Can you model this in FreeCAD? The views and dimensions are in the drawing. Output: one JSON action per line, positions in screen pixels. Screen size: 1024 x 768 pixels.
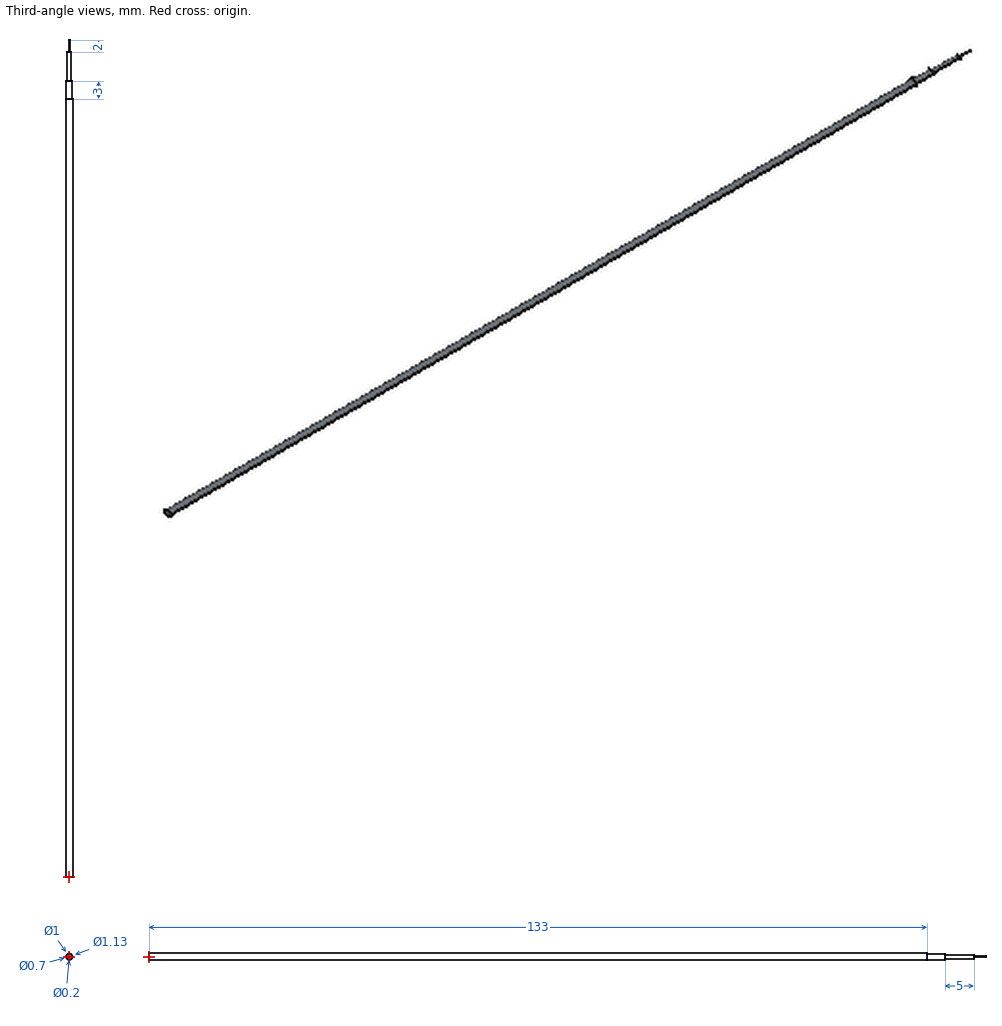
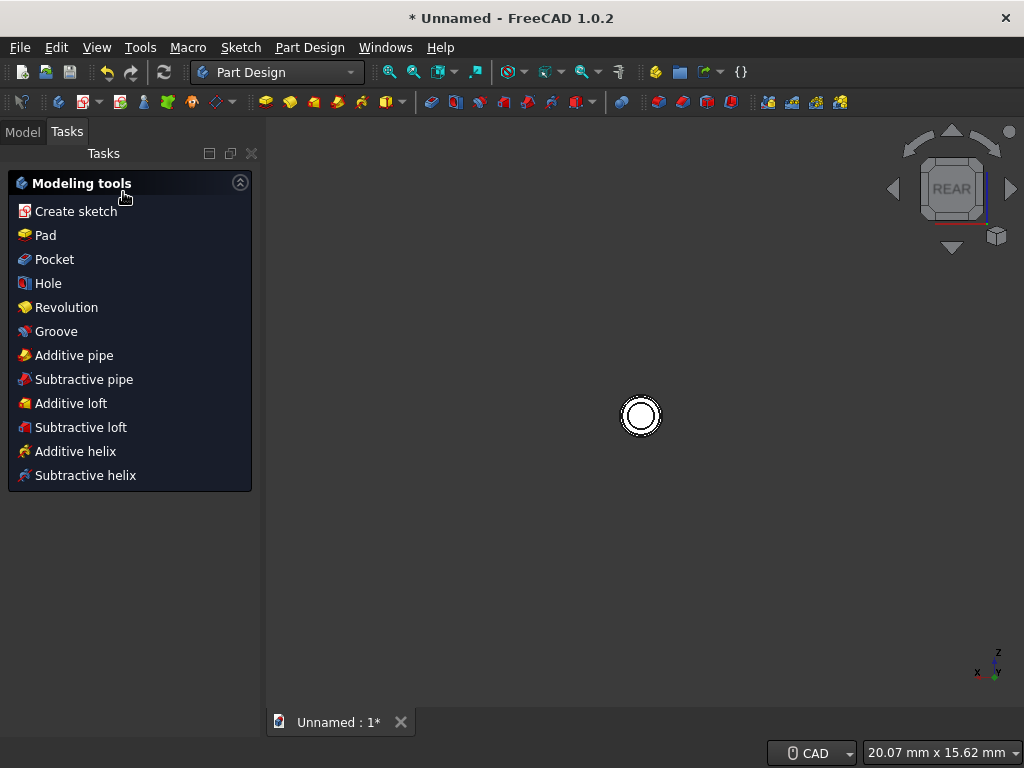
{"action": "left_click", "coordinate": [266, 102]}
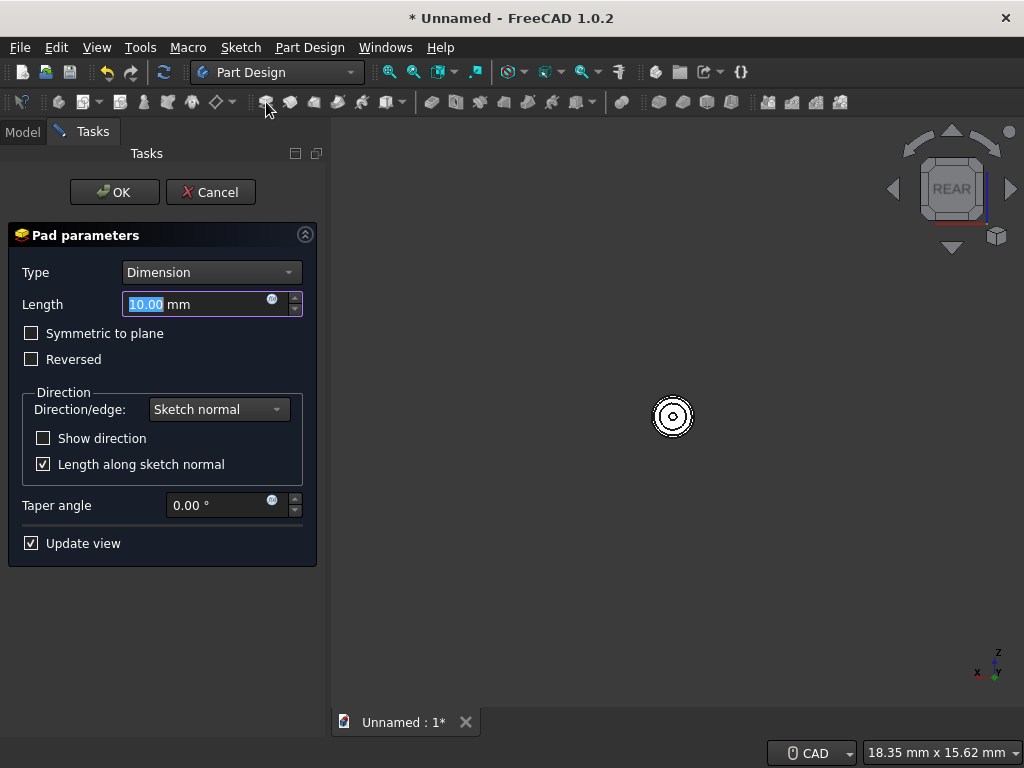
{"action": "type", "text": "2"}
{"action": "key", "text": "Tab"}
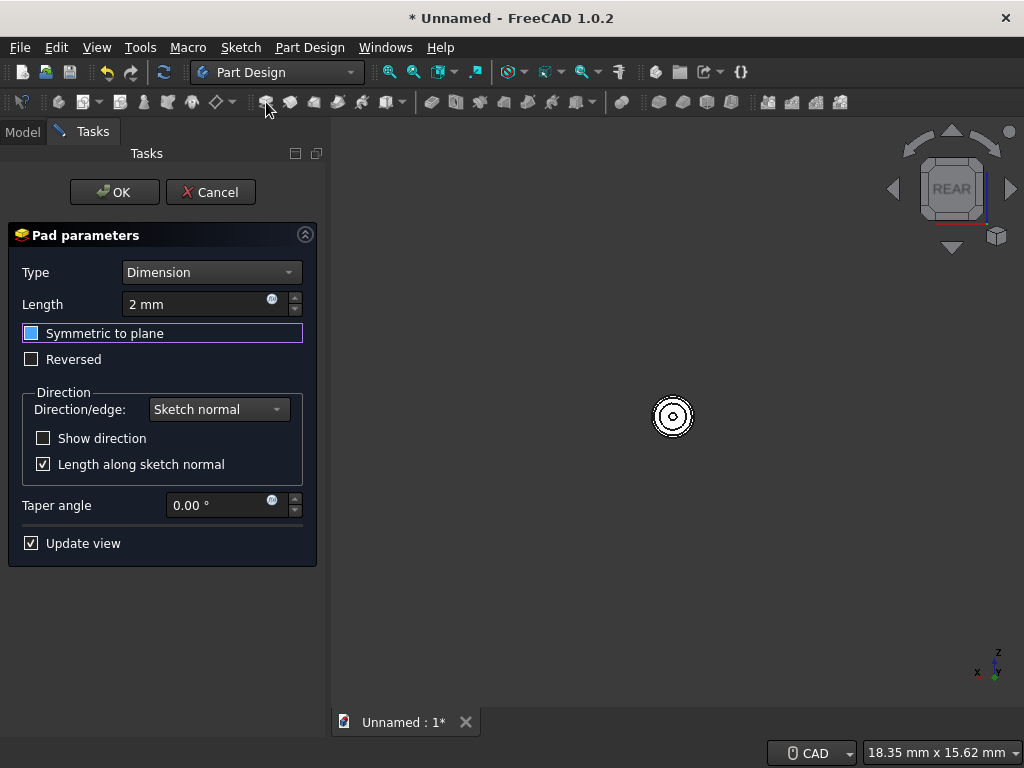
{"action": "left_click", "coordinate": [115, 192]}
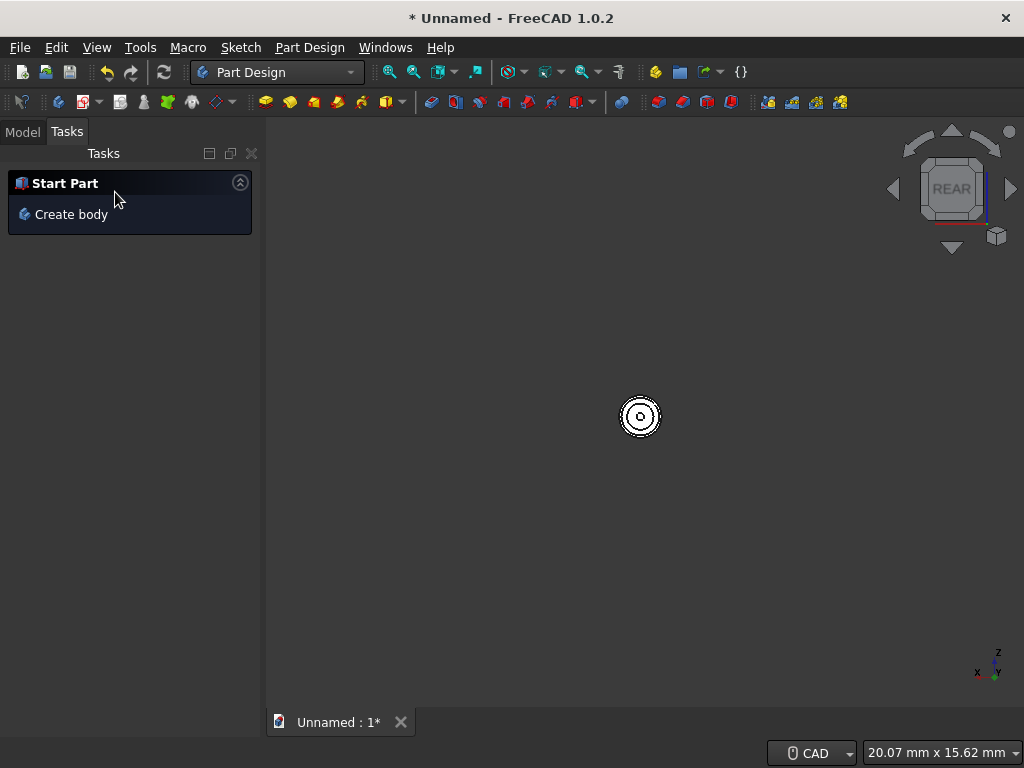
{"action": "key", "text": "0"}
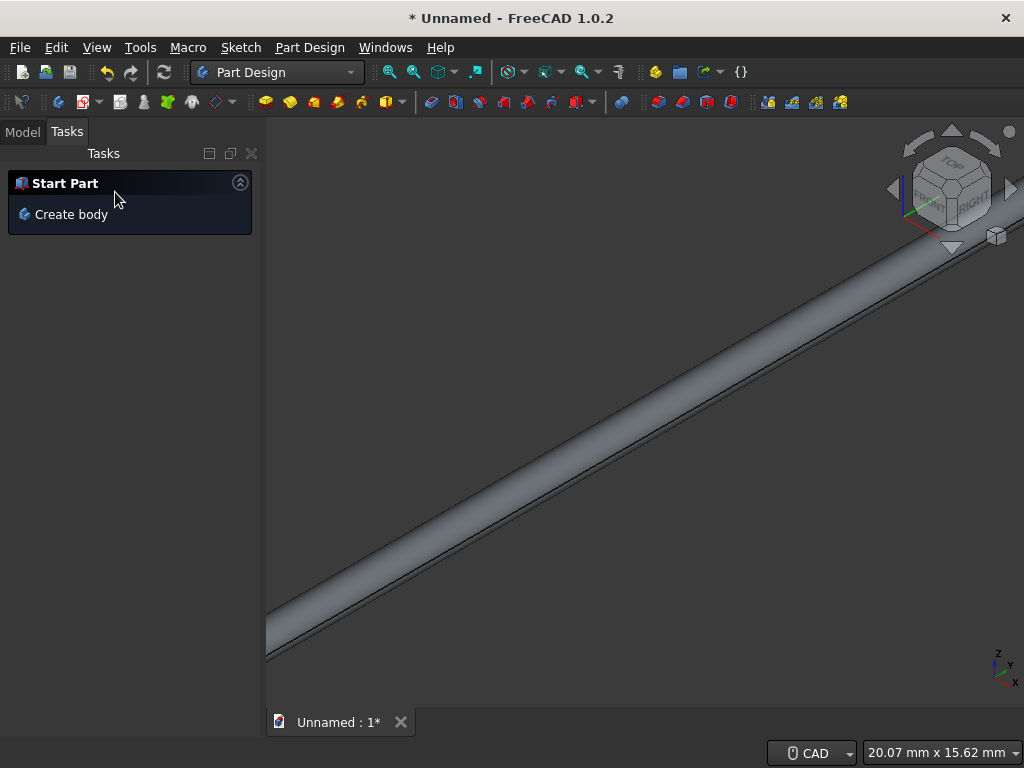
{"action": "left_click", "coordinate": [390, 72]}